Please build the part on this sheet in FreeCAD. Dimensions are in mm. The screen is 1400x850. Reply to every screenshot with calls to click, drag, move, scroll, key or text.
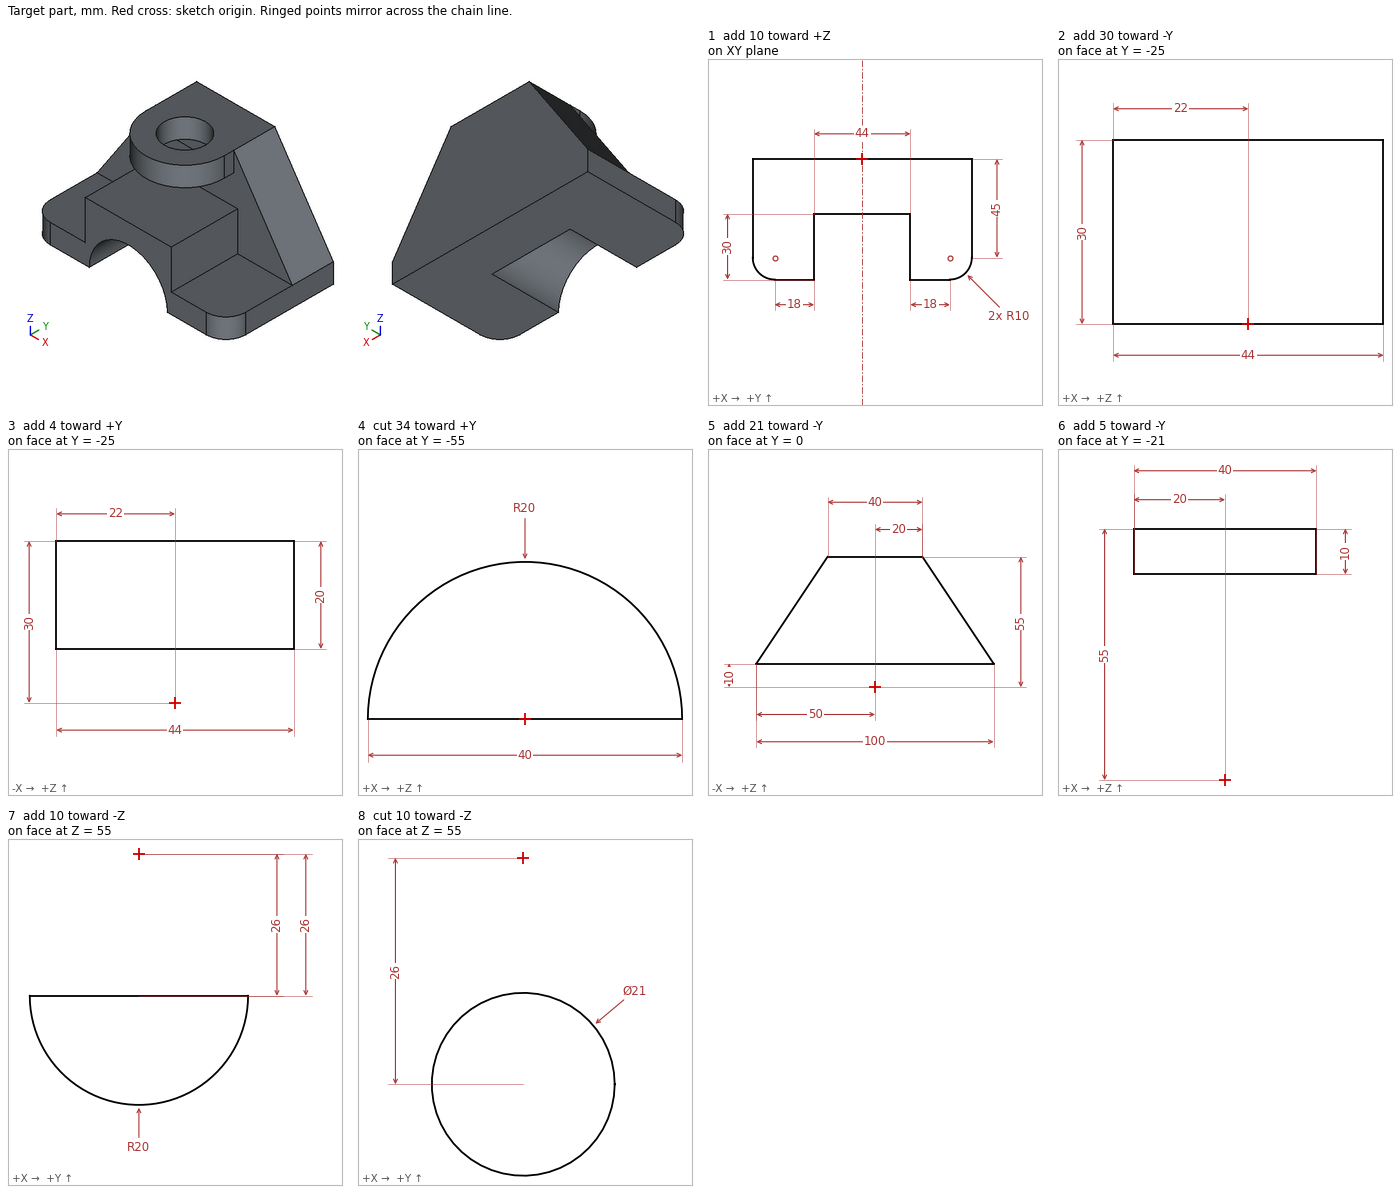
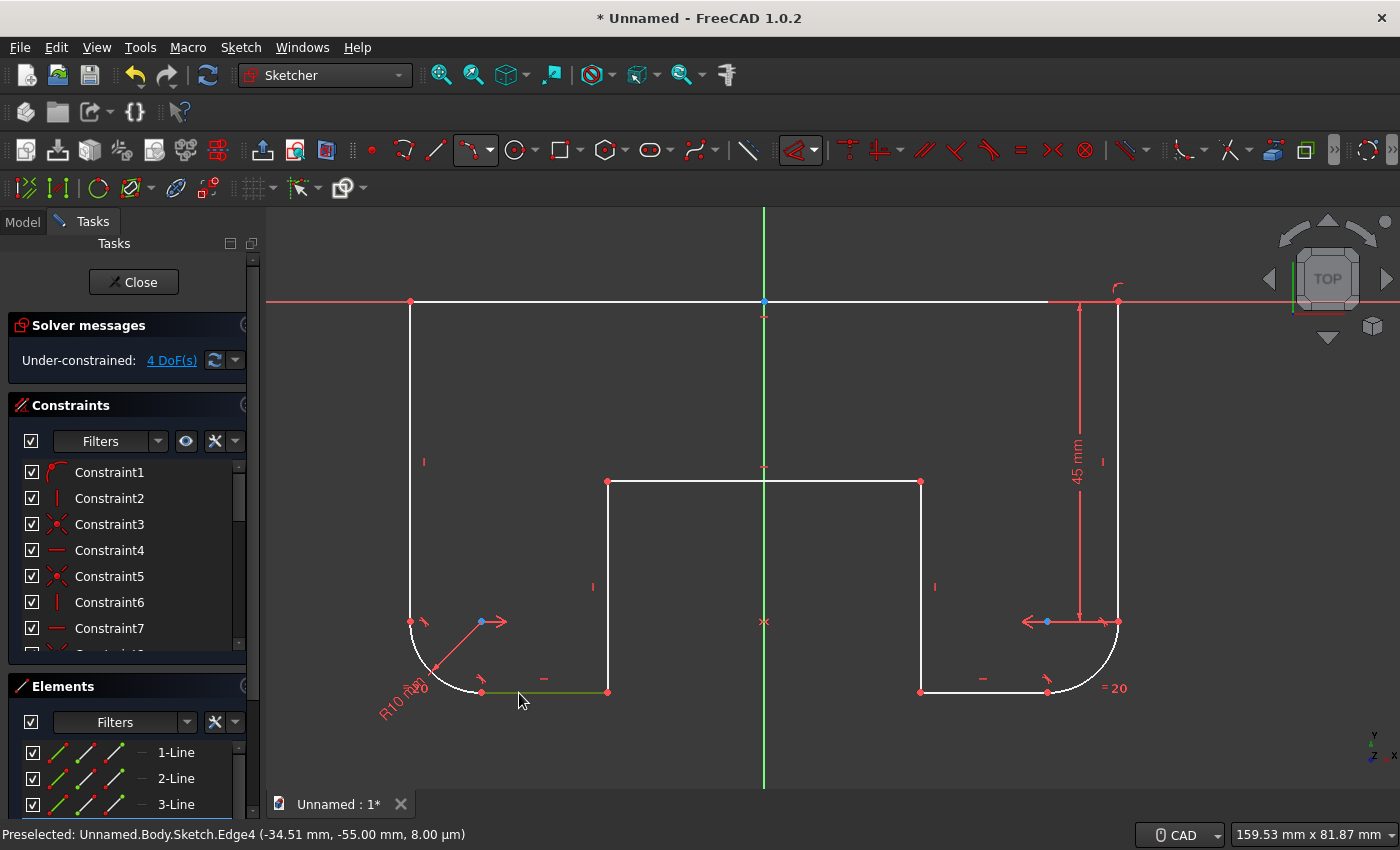
key(l)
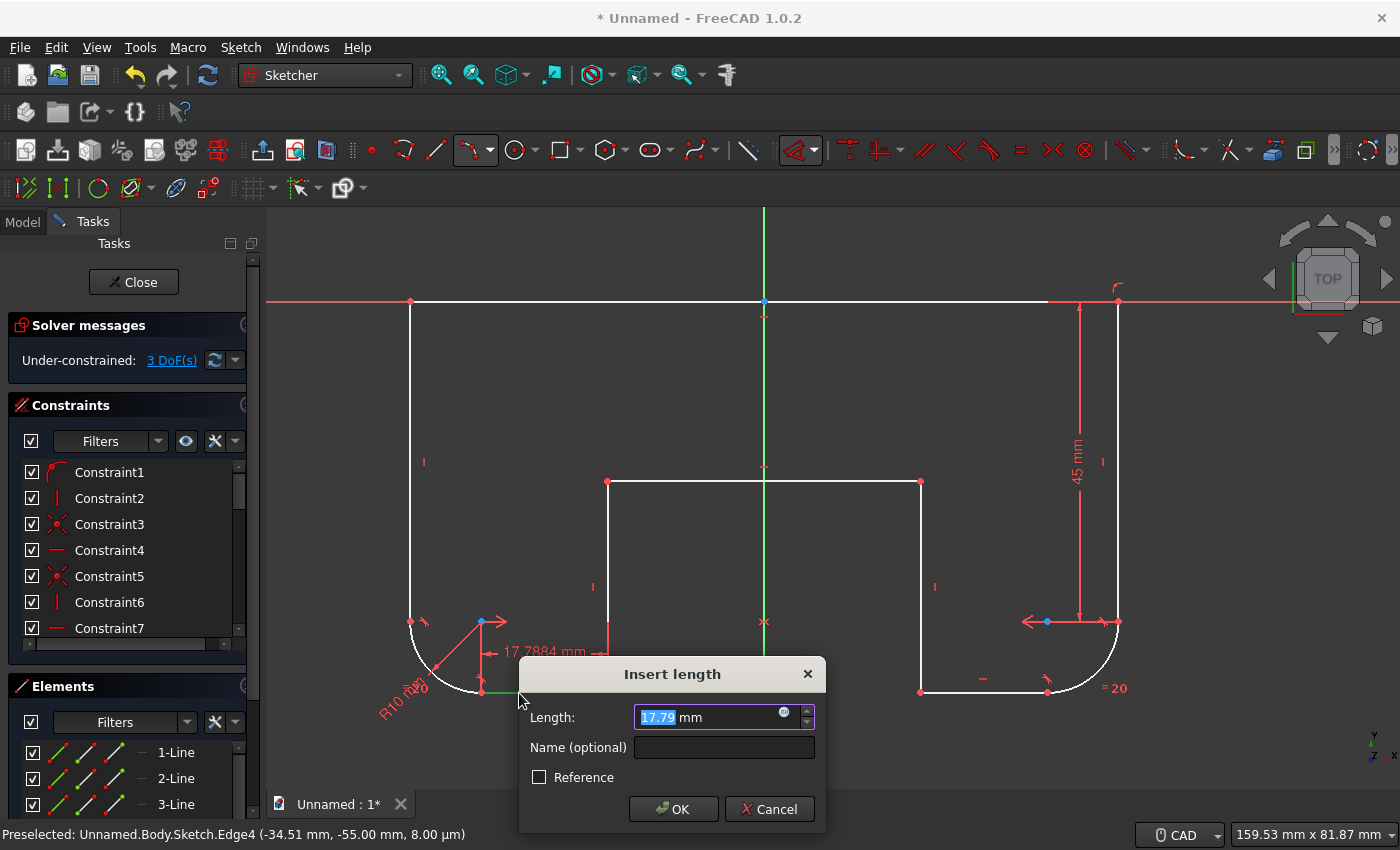
text(18)
key(Return)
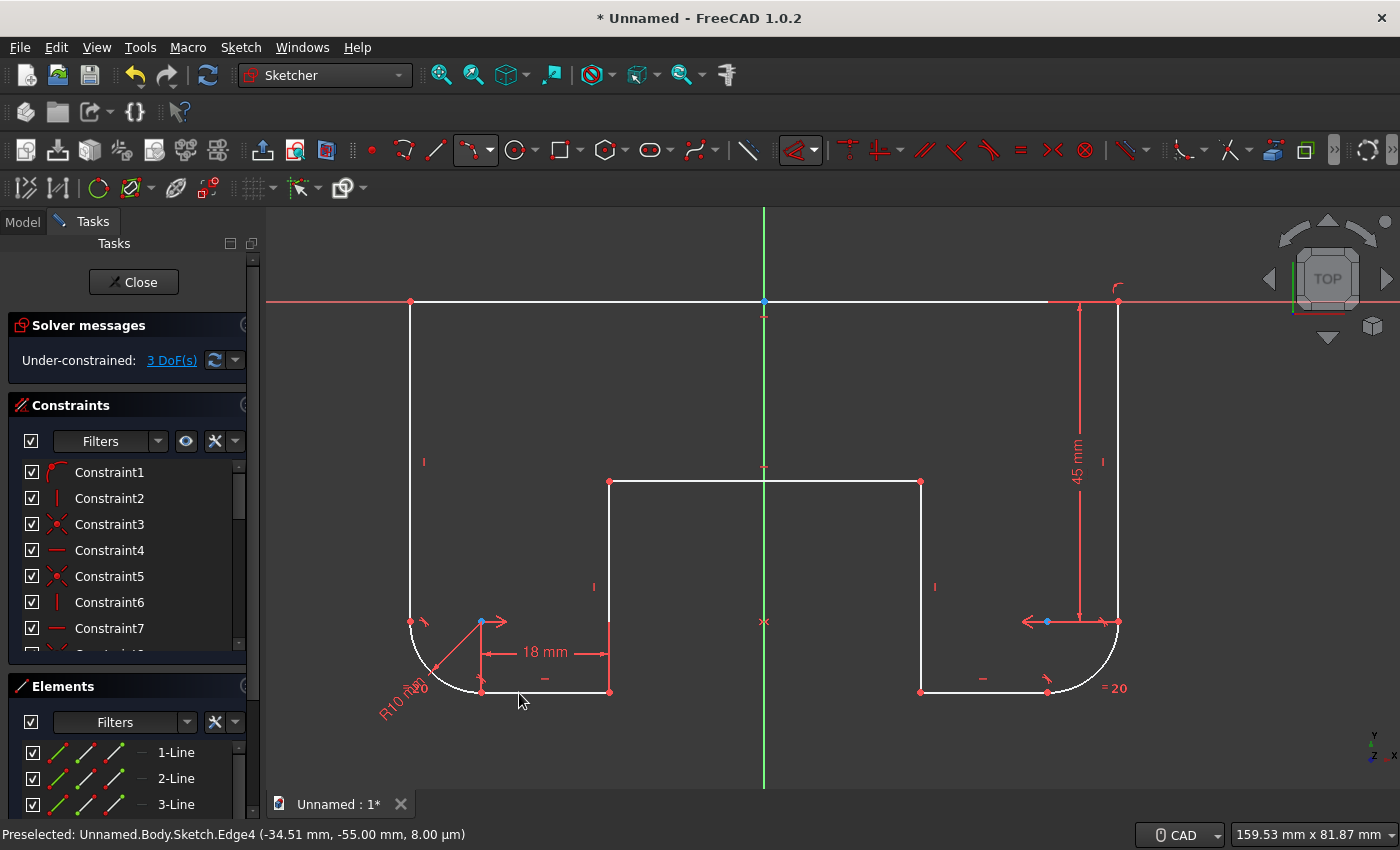
click(609, 629)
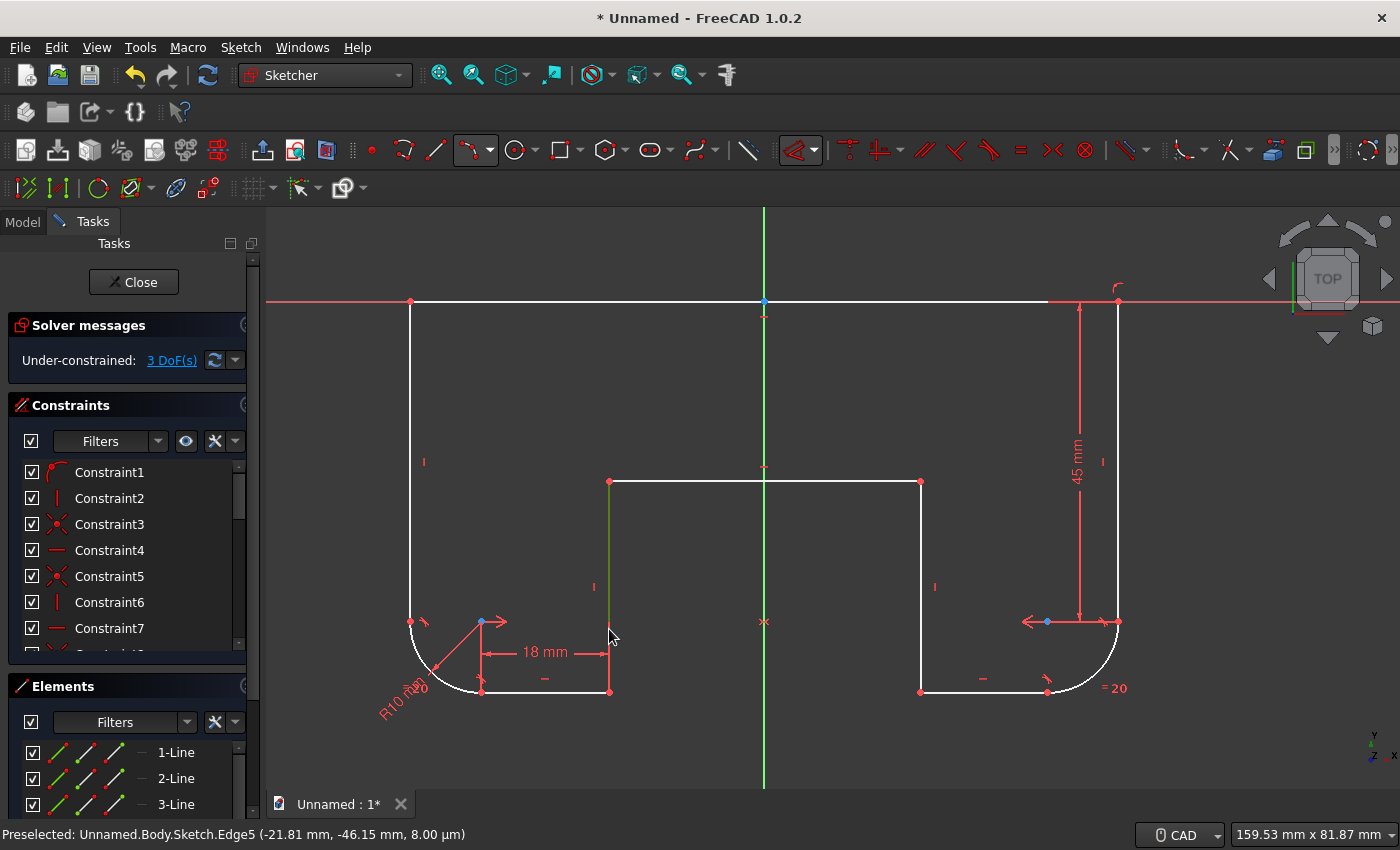
key(i)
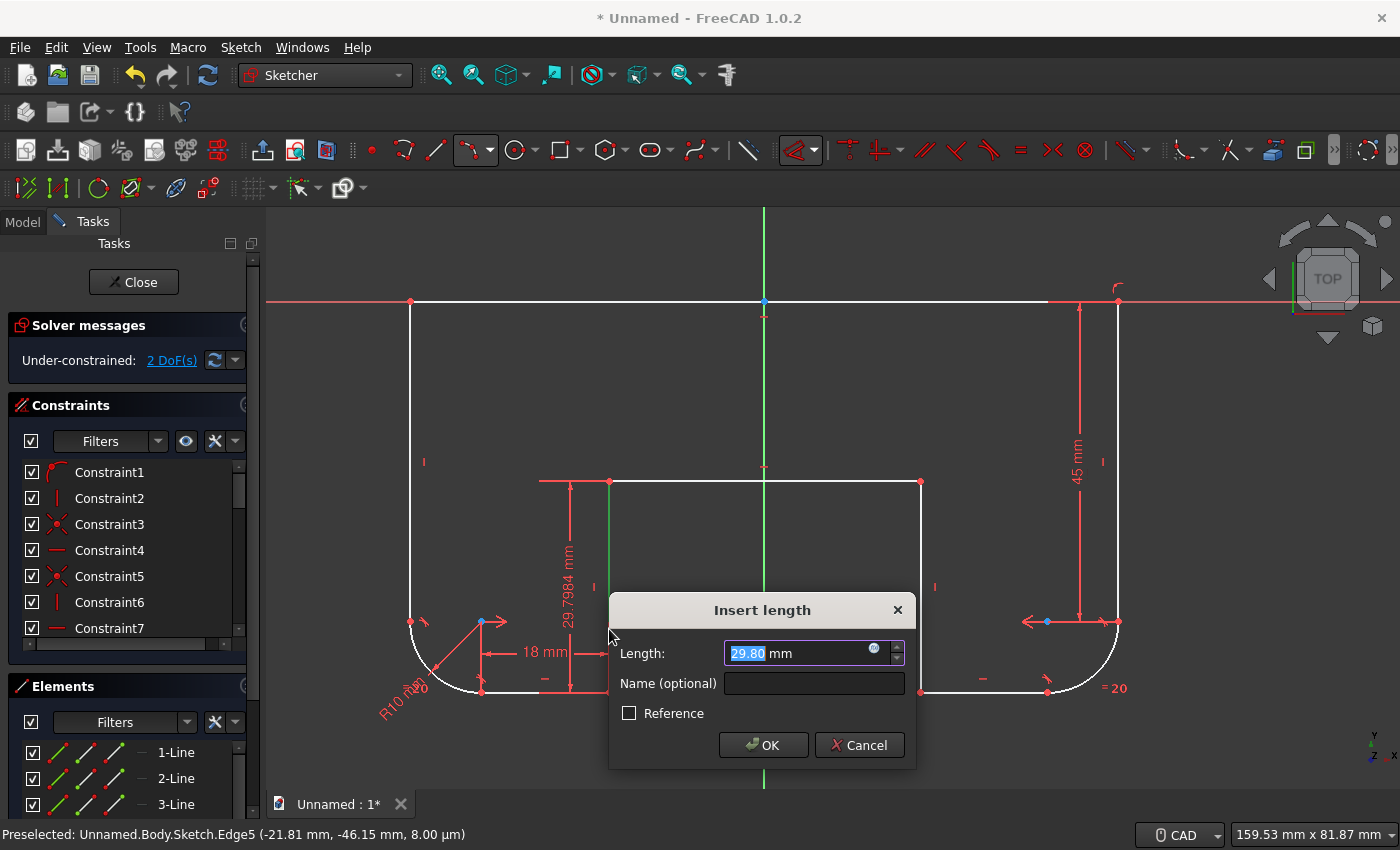
text(30)
key(Return)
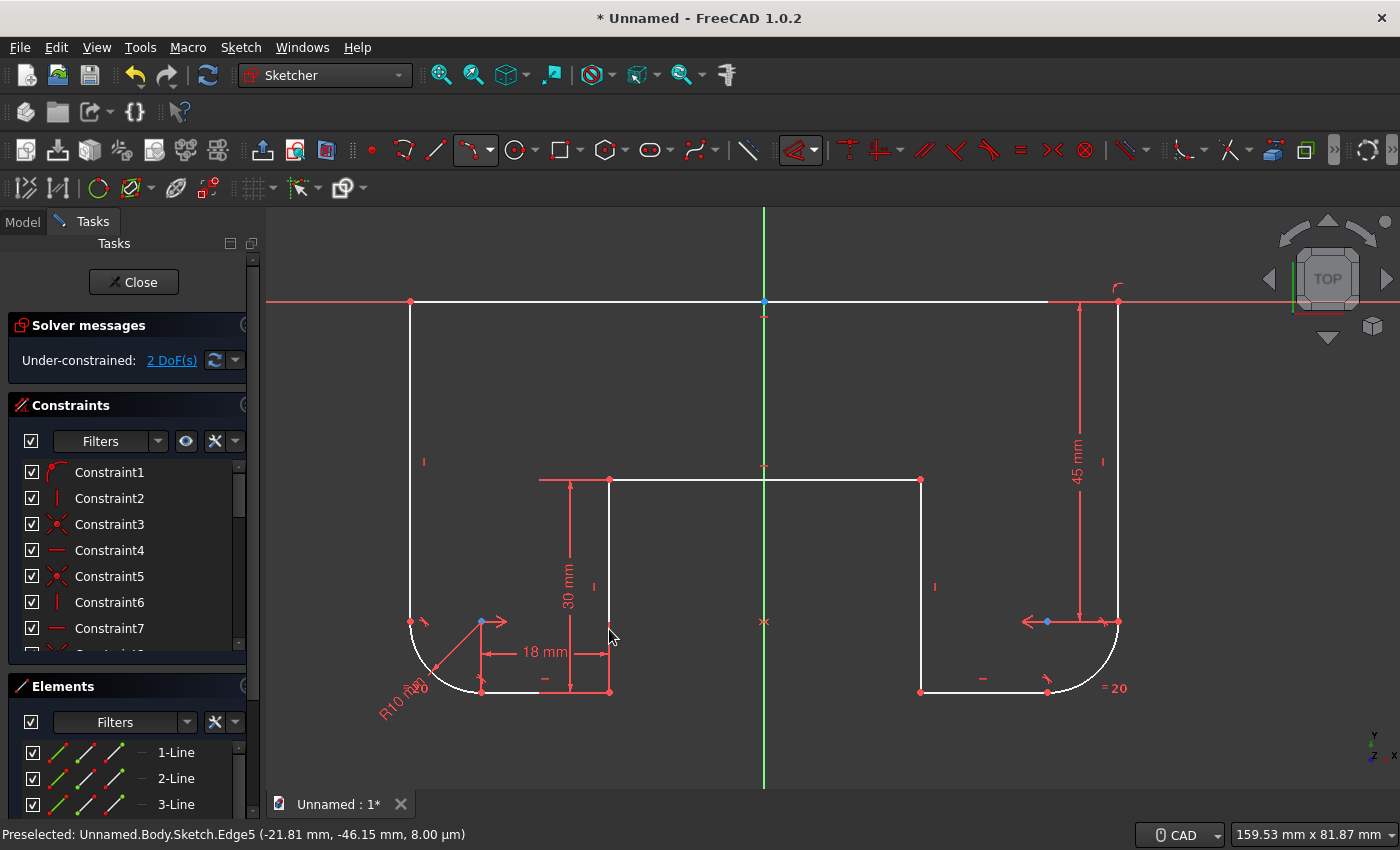
click(703, 480)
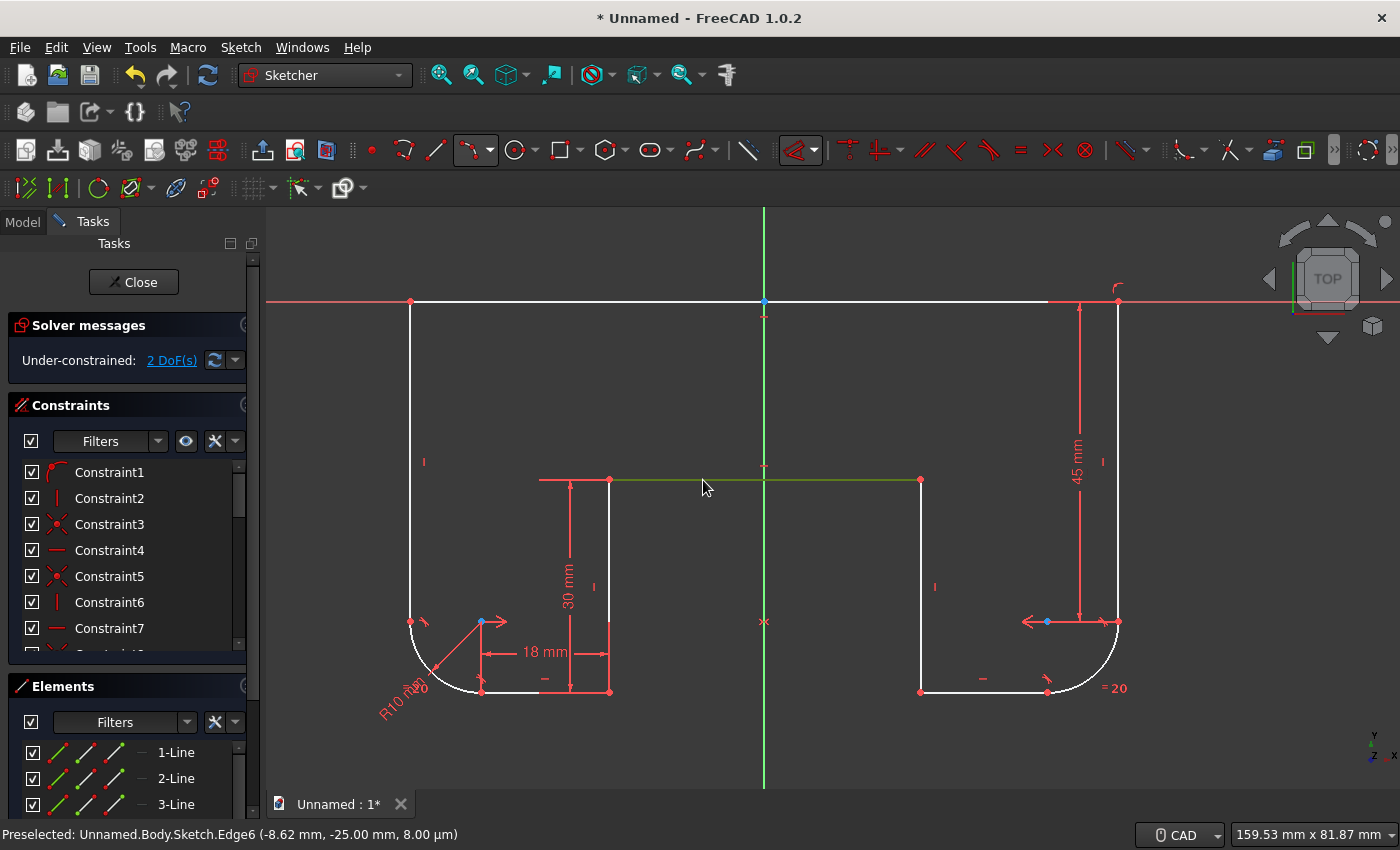
key(l)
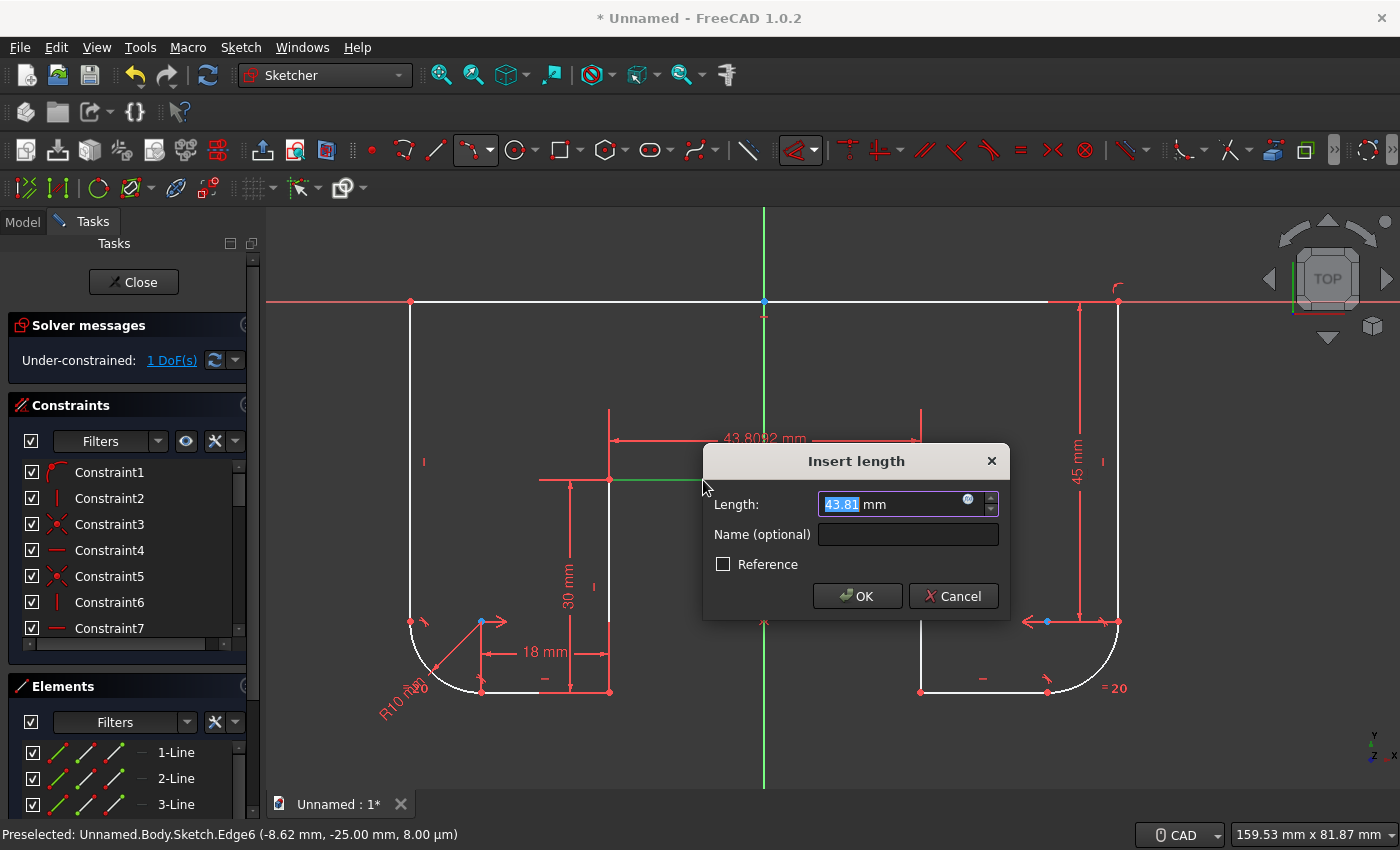
text(44)
key(Return)